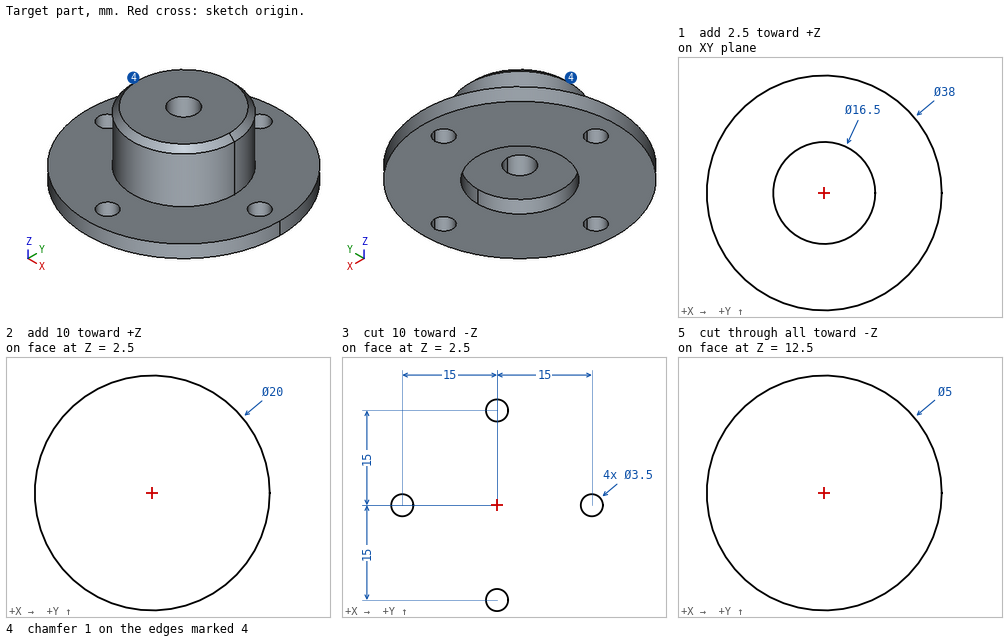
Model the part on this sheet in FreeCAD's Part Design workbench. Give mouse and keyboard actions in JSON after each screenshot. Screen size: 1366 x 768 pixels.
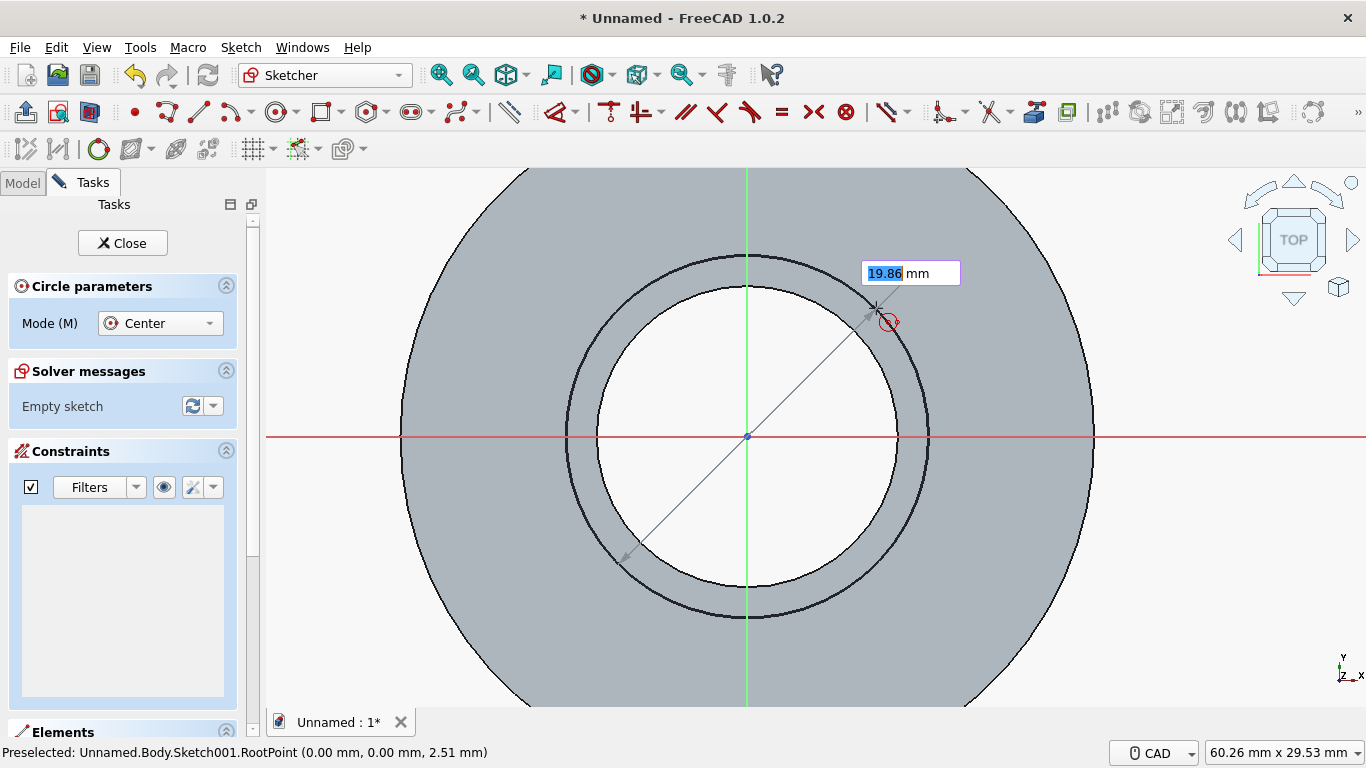
{"action": "type", "text": "20"}
{"action": "key", "text": "Return"}
{"action": "key", "text": "Escape"}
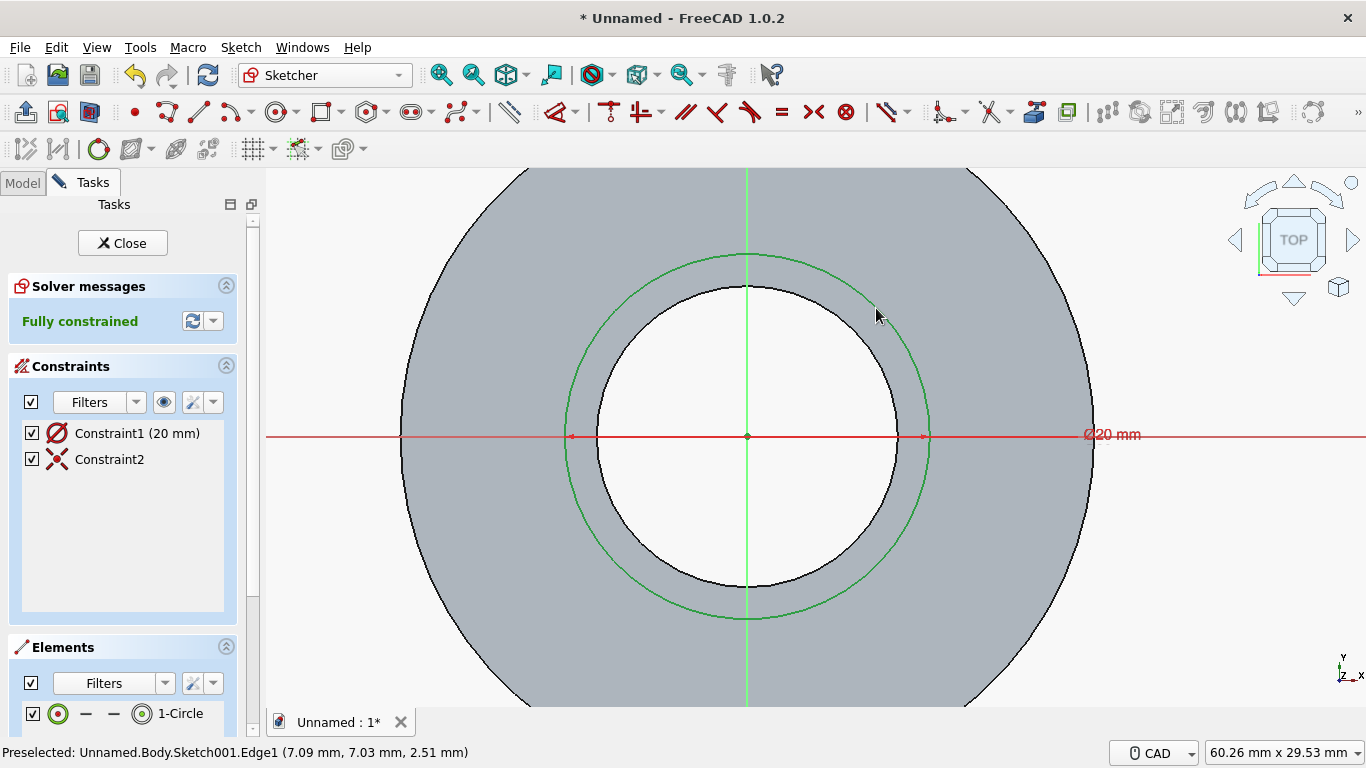
{"action": "left_click", "coordinate": [123, 243]}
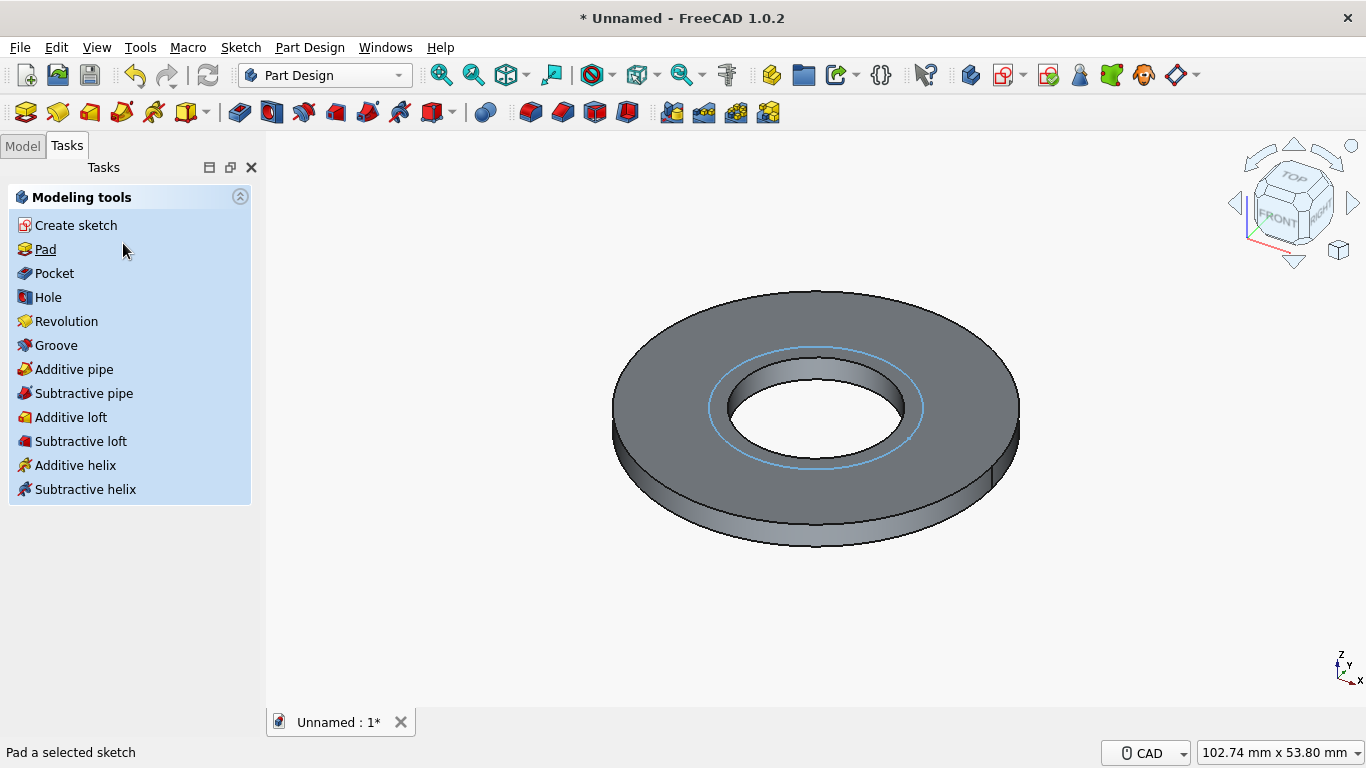
{"action": "left_click", "coordinate": [26, 112]}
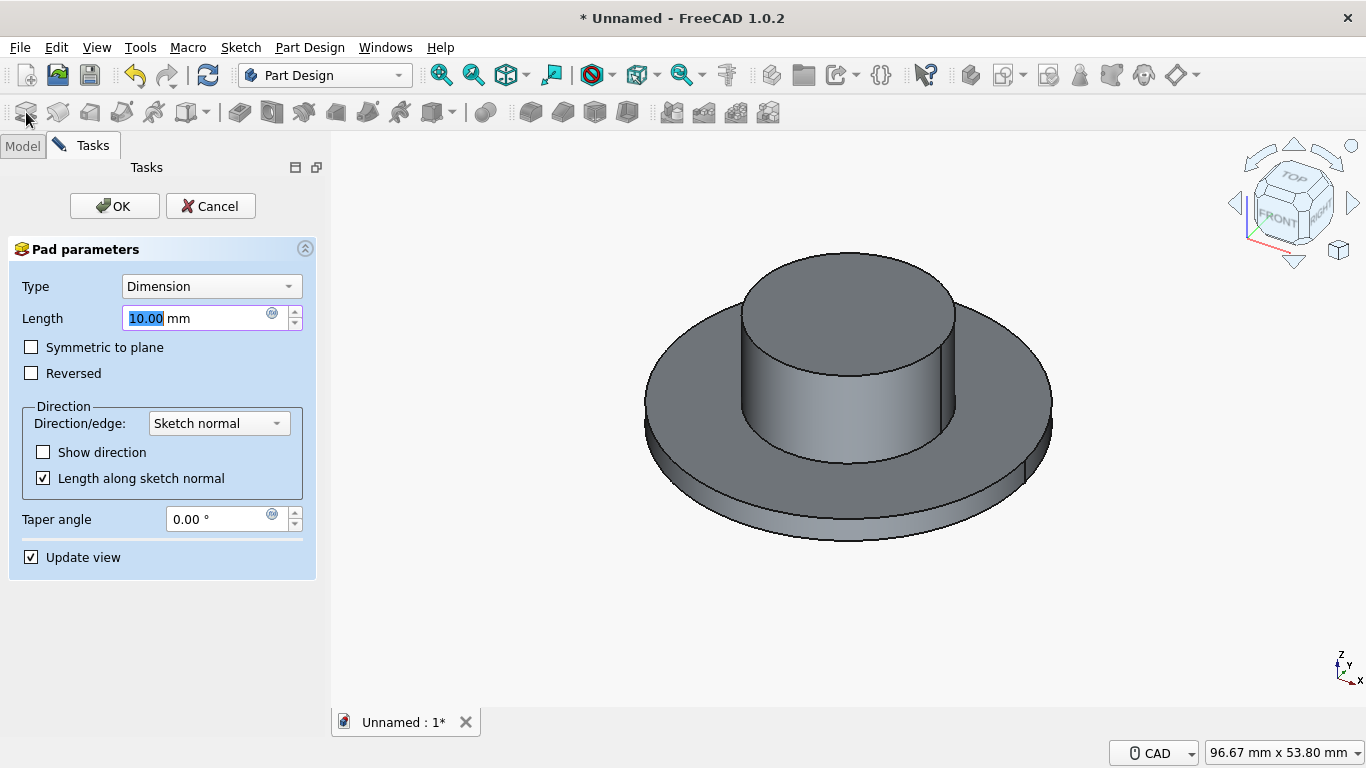
{"action": "type", "text": "10"}
{"action": "key", "text": "Tab"}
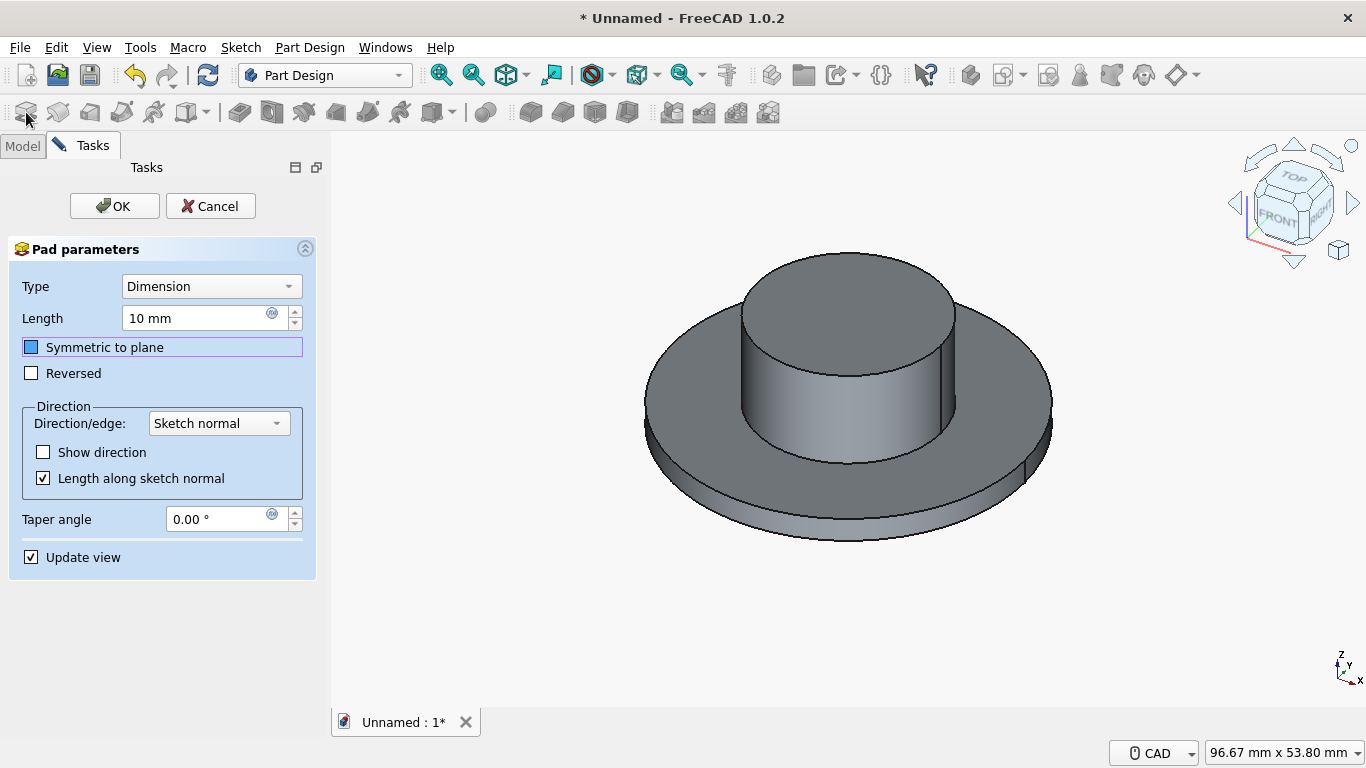
{"action": "left_click", "coordinate": [115, 206]}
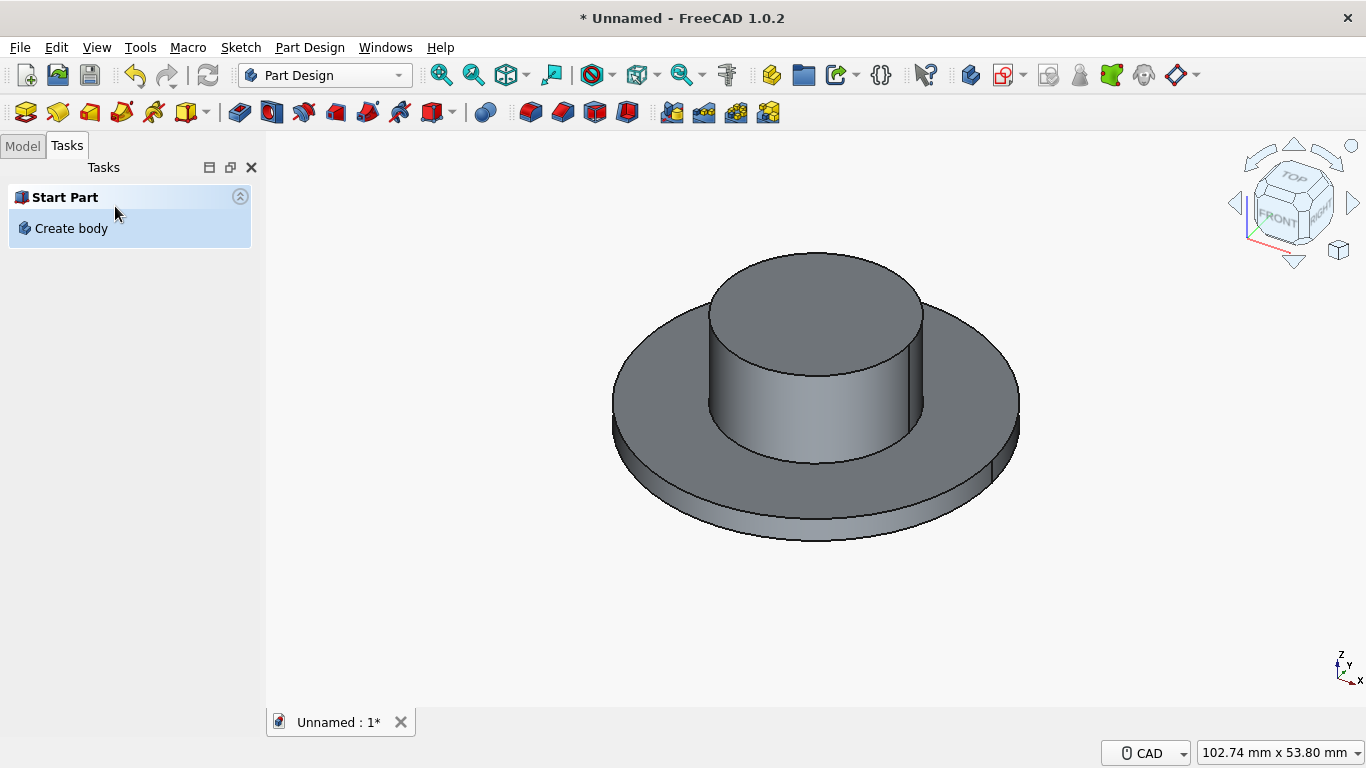
{"action": "left_click", "coordinate": [859, 492]}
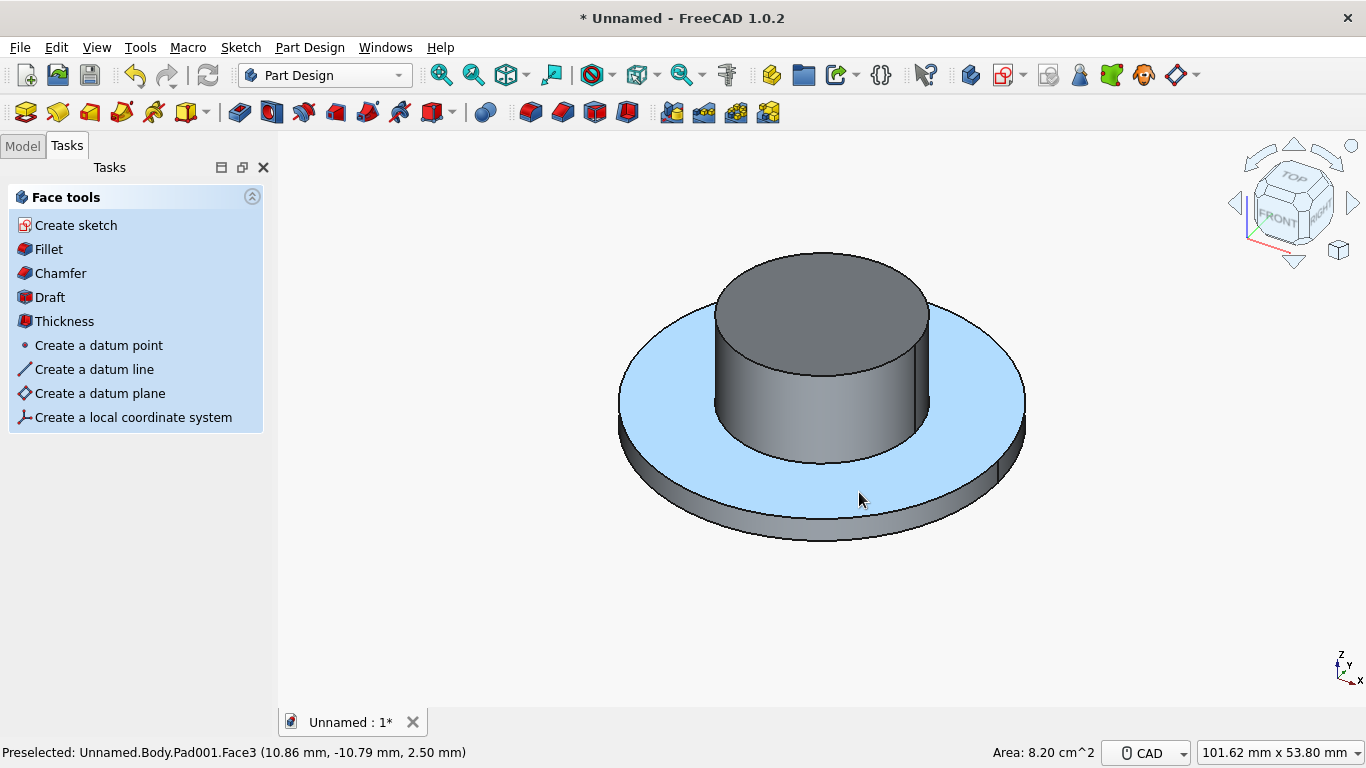
{"action": "left_click", "coordinate": [1004, 76]}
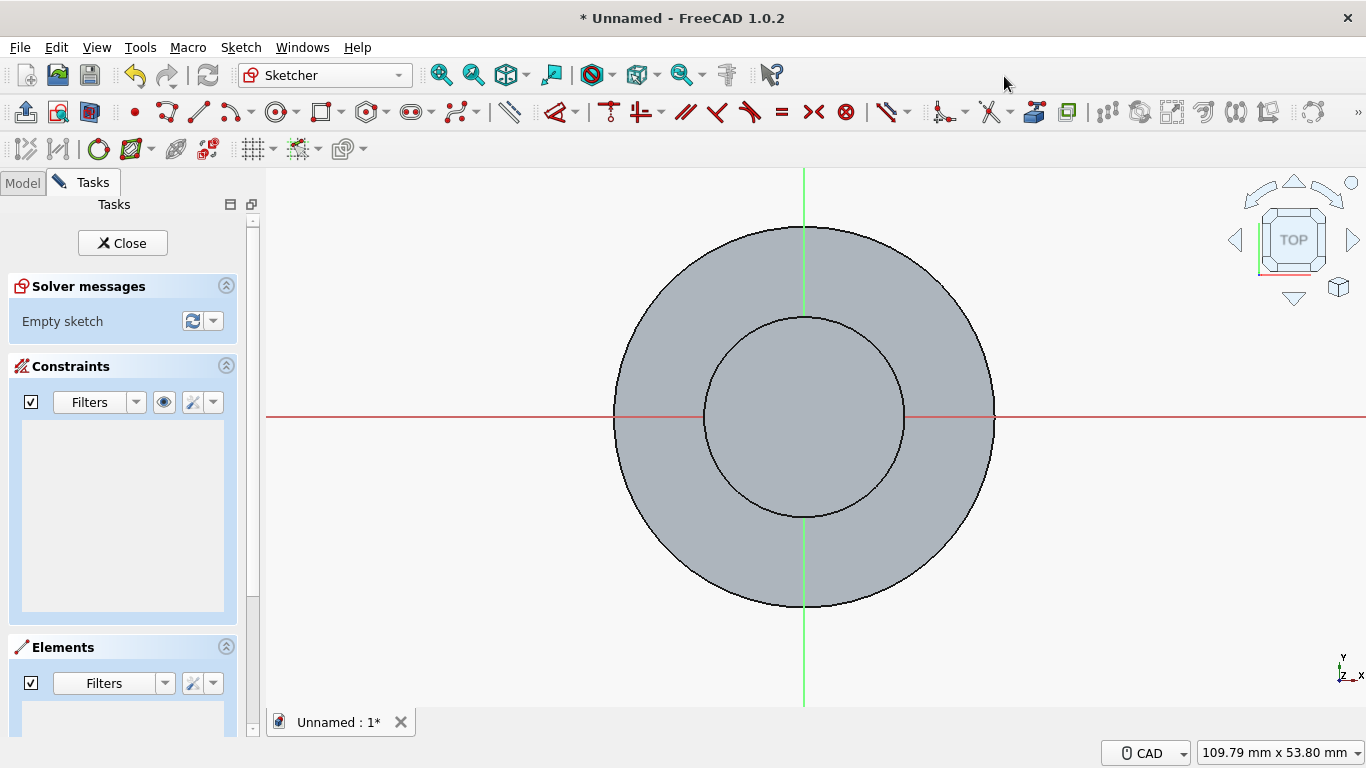
{"action": "left_click", "coordinate": [90, 112]}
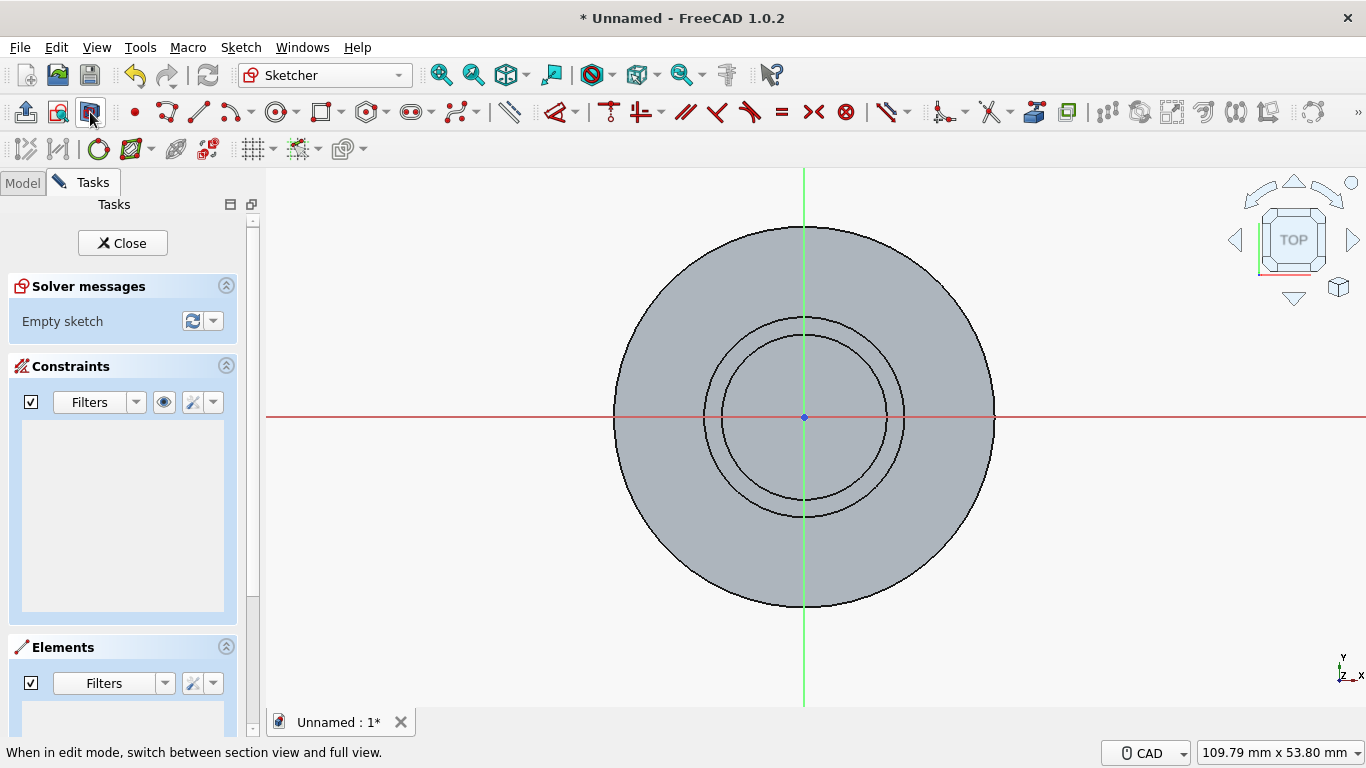
{"action": "key", "text": "g c"}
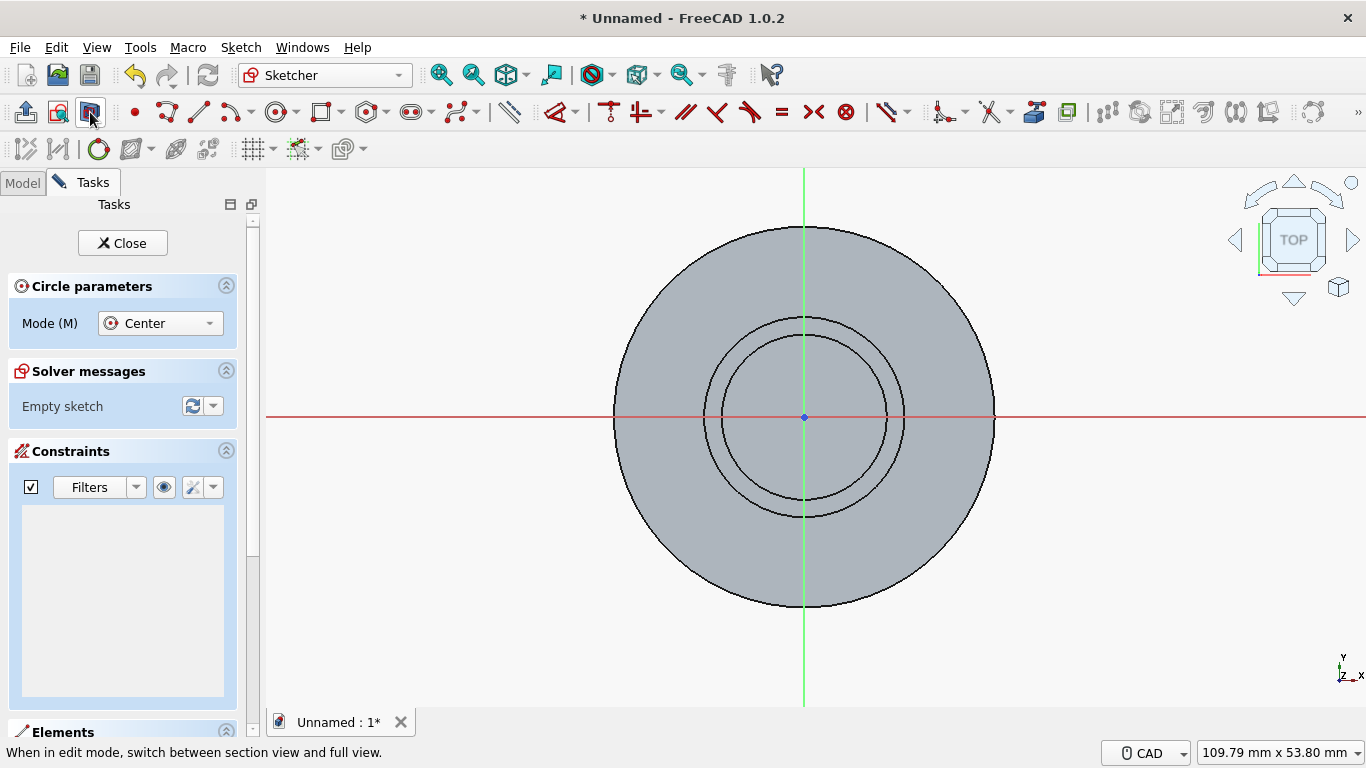
{"action": "scroll", "coordinate": [955, 417], "scroll_direction": "up", "scroll_amount": 2}